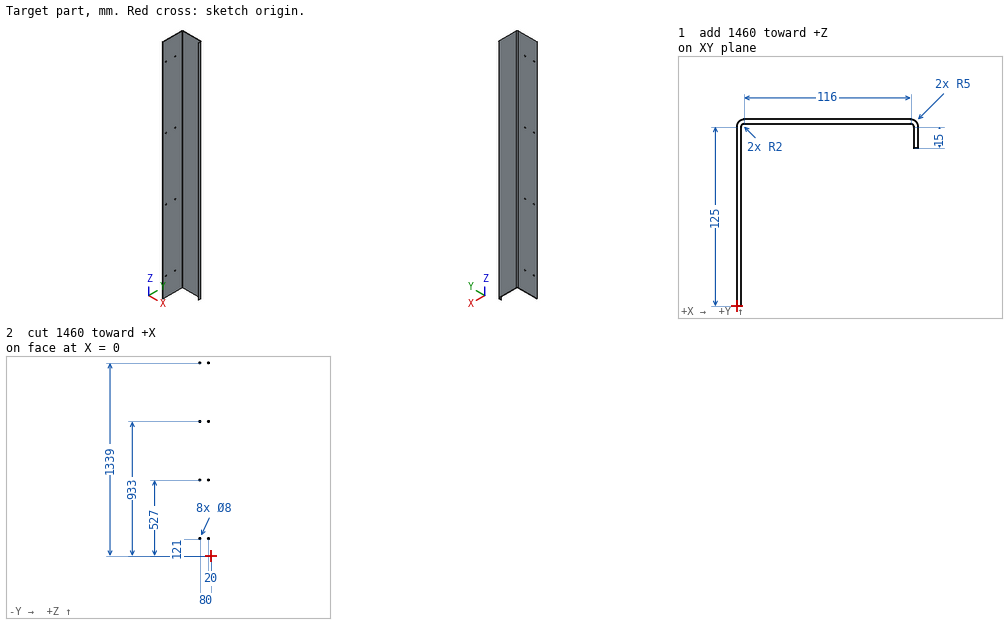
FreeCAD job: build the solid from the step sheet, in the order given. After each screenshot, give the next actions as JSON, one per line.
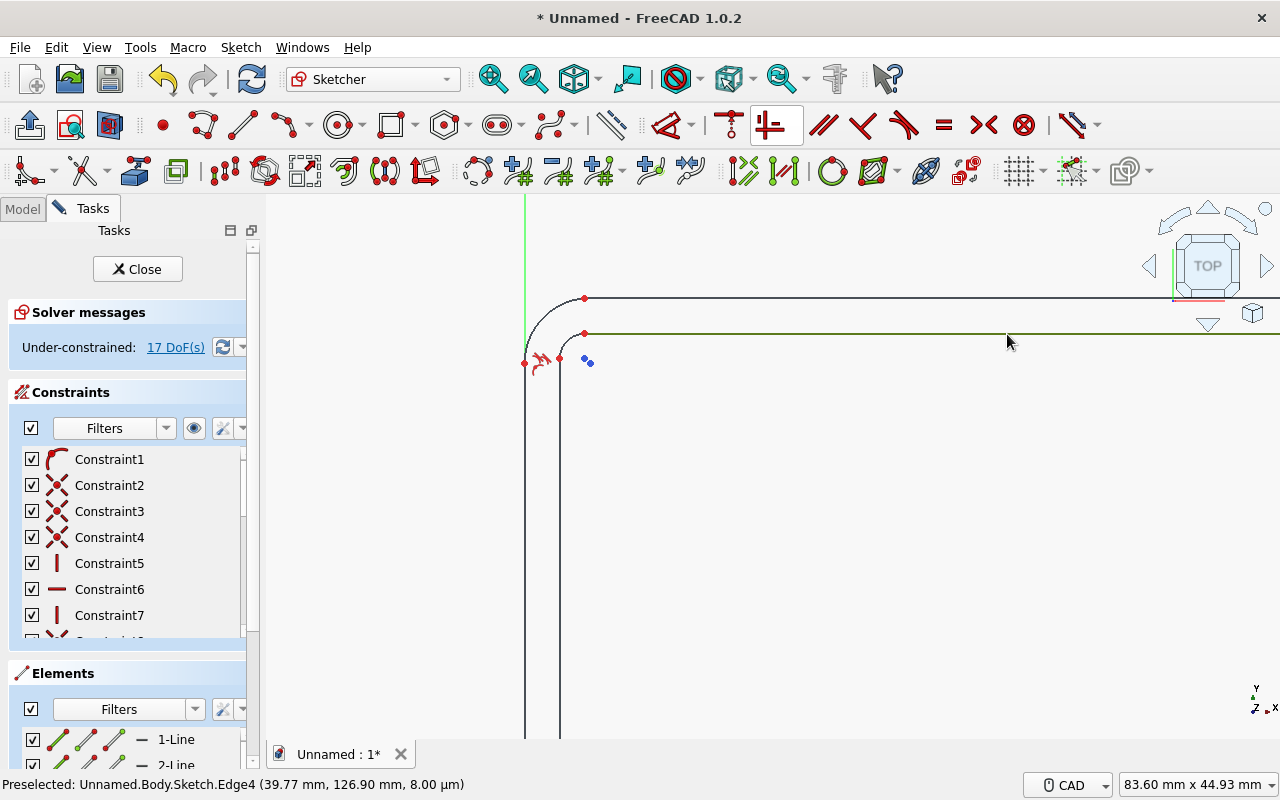
{"action": "left_click", "coordinate": [573, 337]}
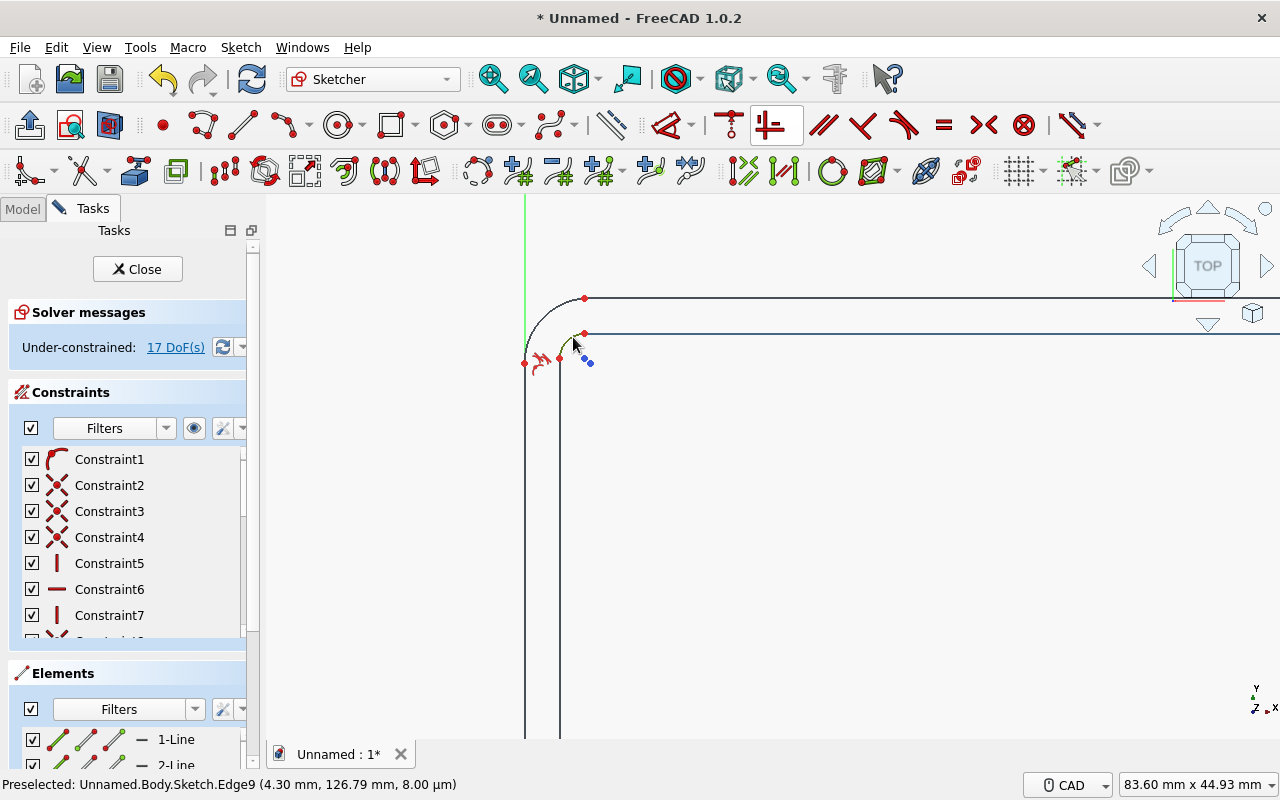
{"action": "left_click", "coordinate": [904, 126]}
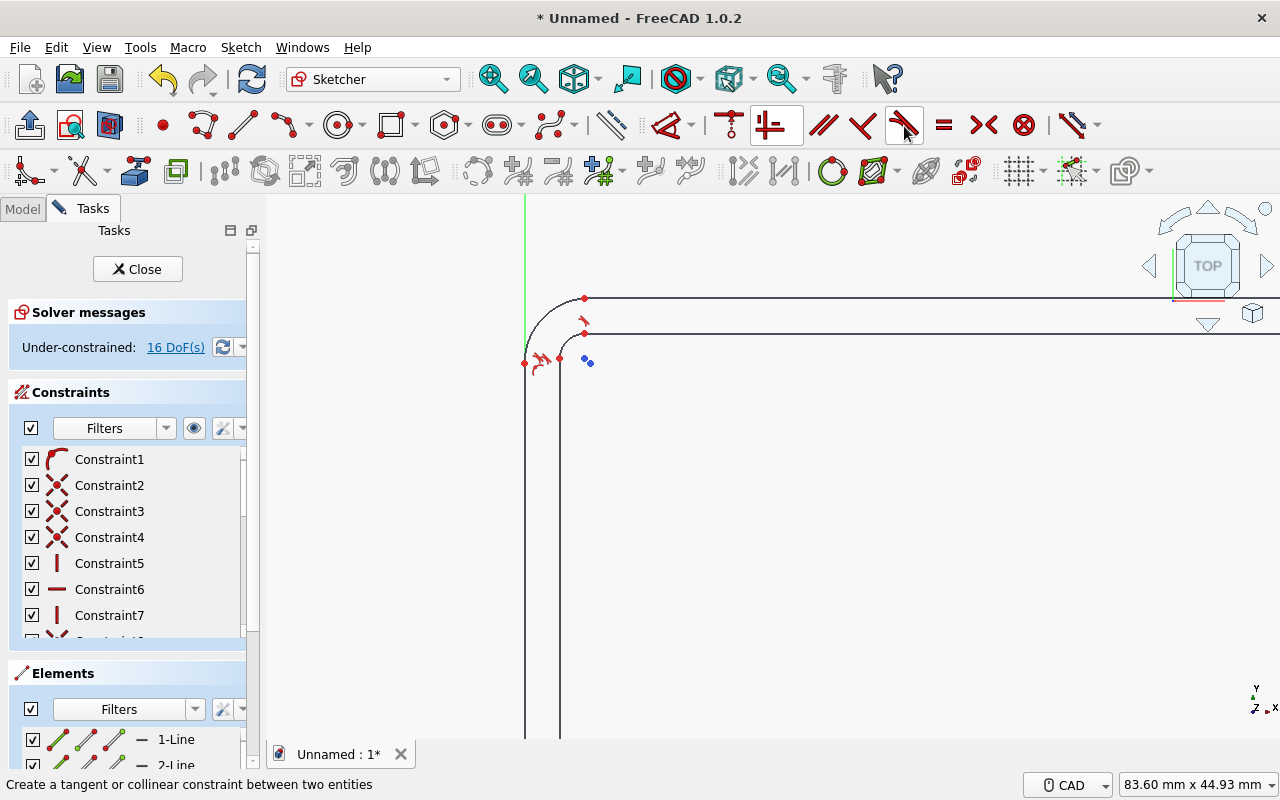
{"action": "left_click", "coordinate": [1007, 334]}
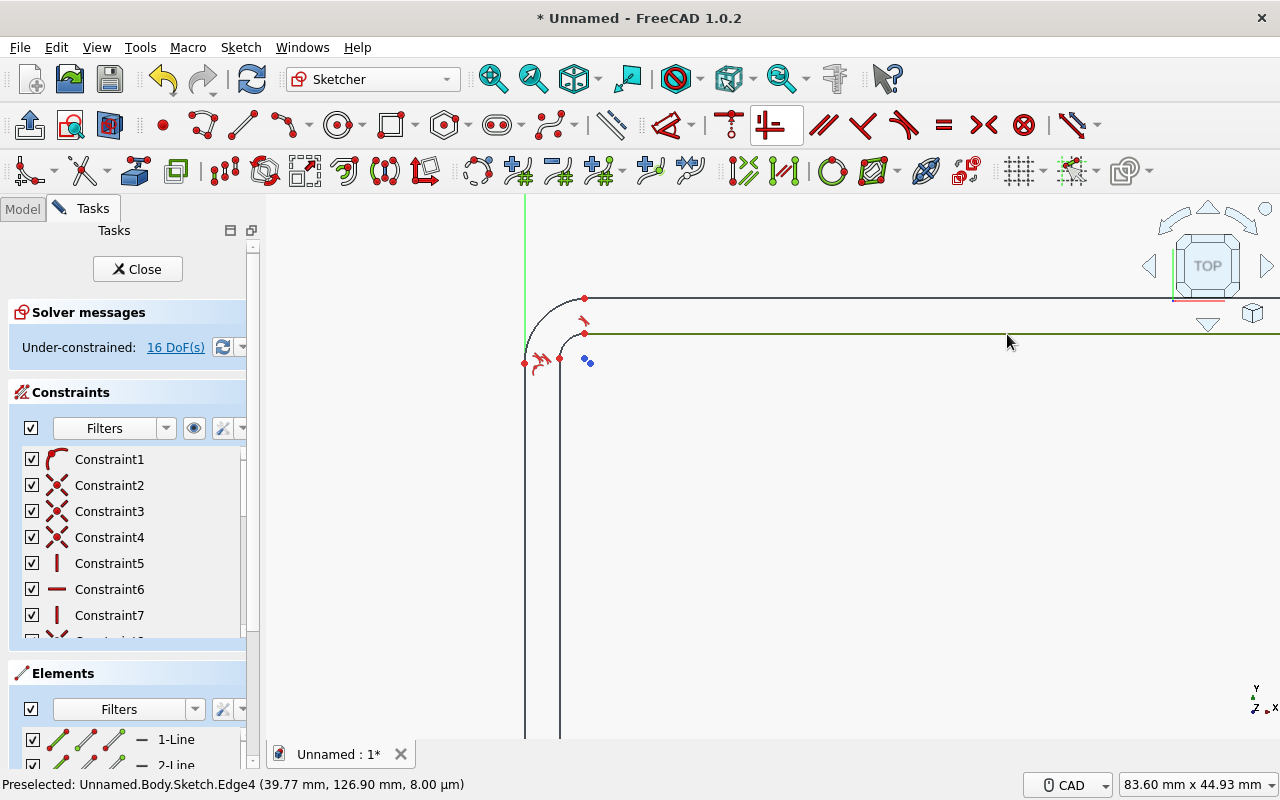
{"action": "scroll", "coordinate": [557, 310], "scroll_direction": "down", "scroll_amount": 8}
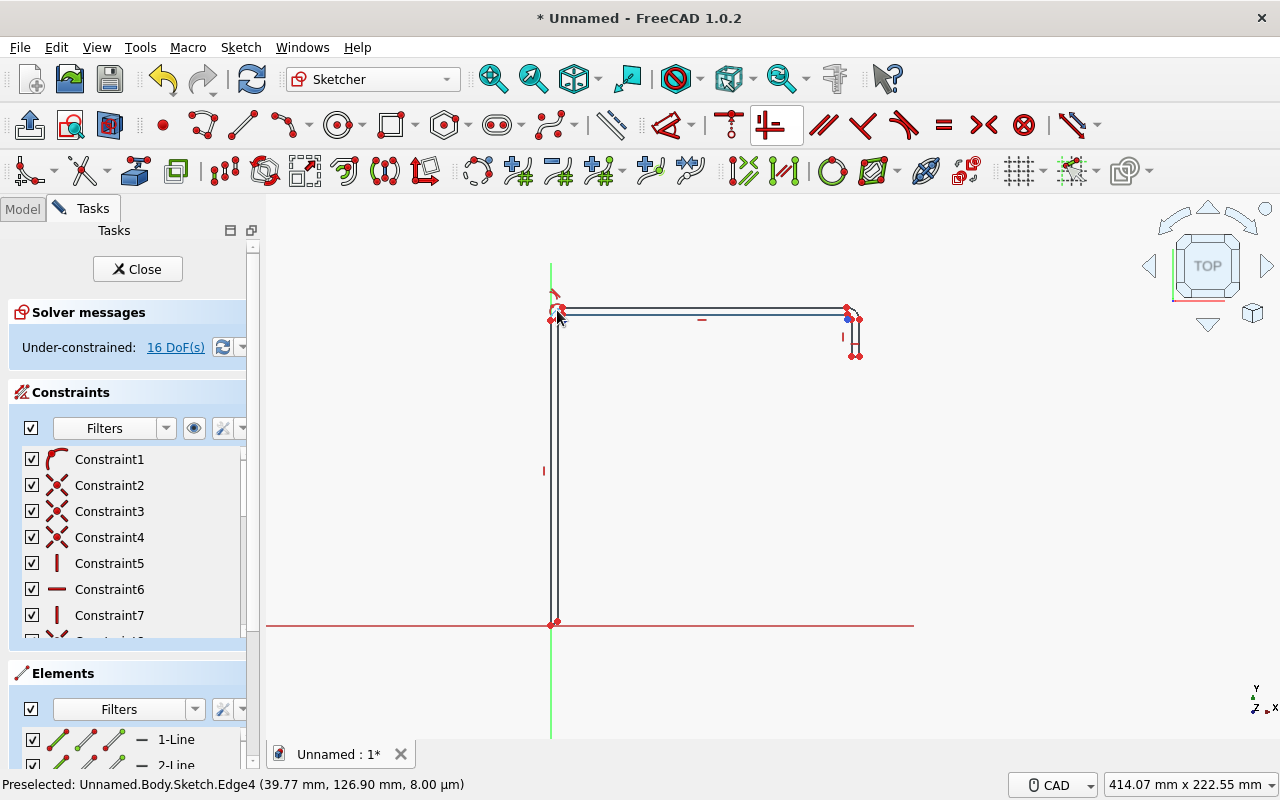
{"action": "scroll", "coordinate": [851, 318], "scroll_direction": "up", "scroll_amount": 9}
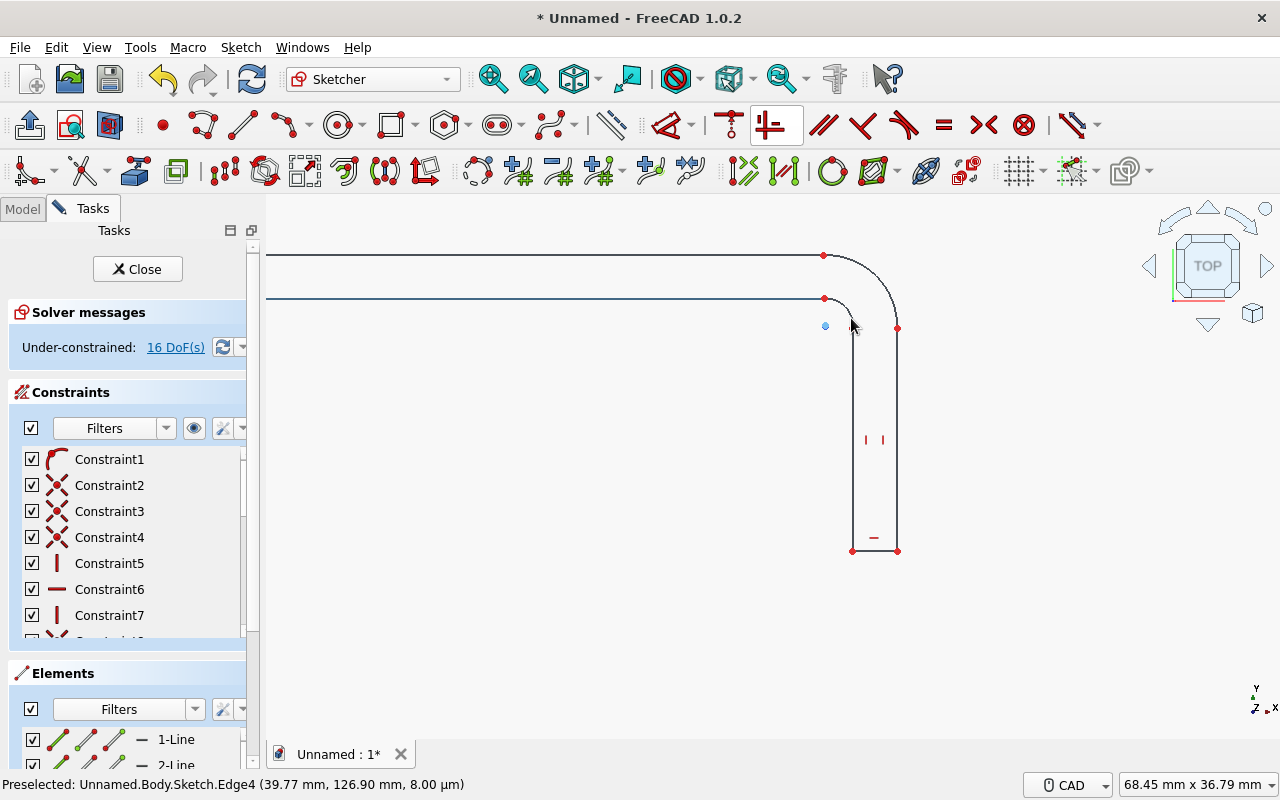
{"action": "left_click", "coordinate": [851, 315]}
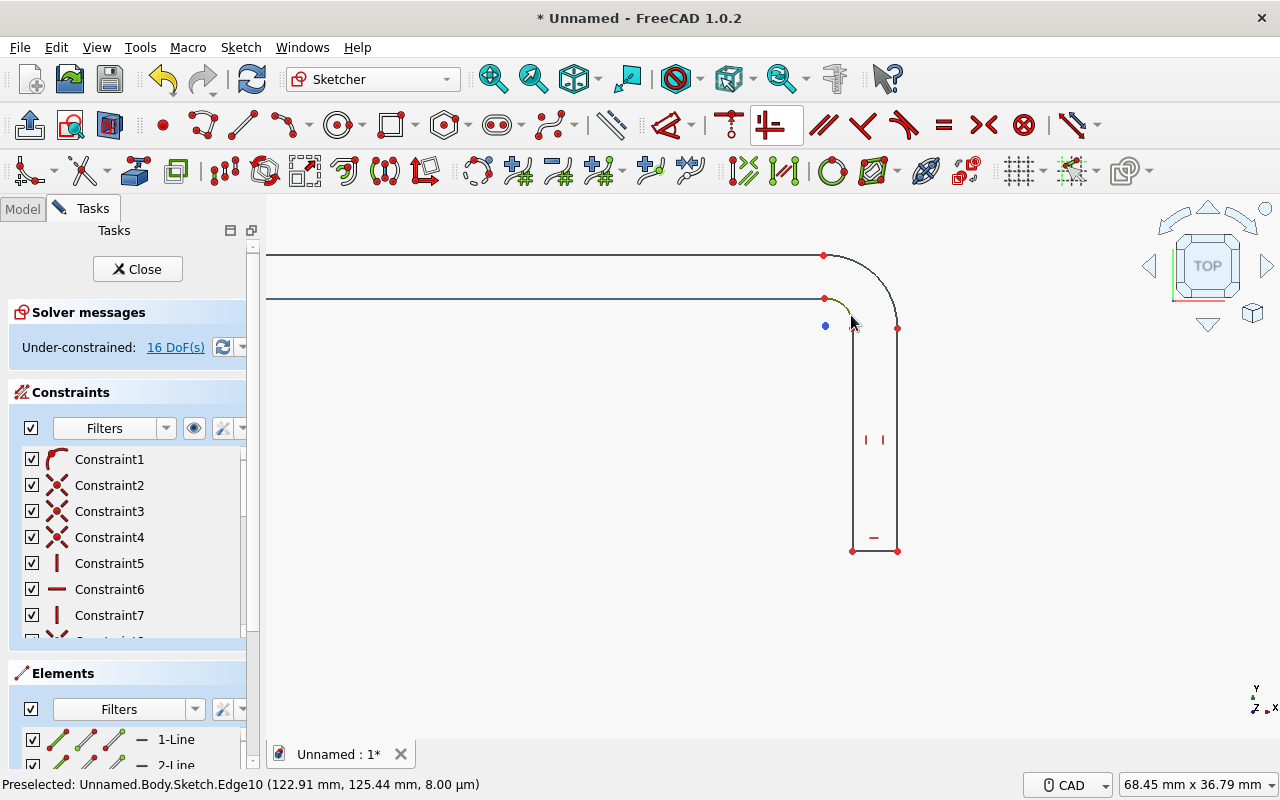
{"action": "left_click", "coordinate": [904, 126]}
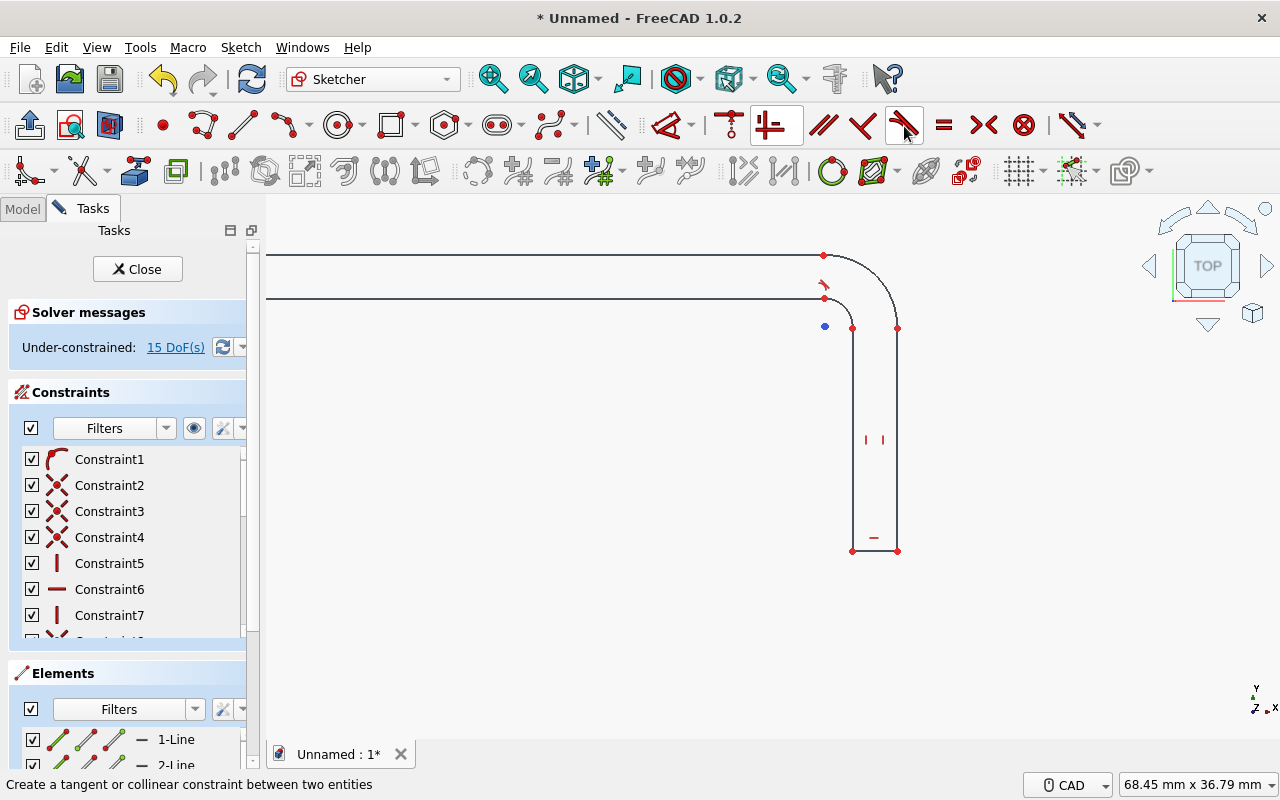
{"action": "scroll", "coordinate": [851, 318], "scroll_direction": "down", "scroll_amount": 9}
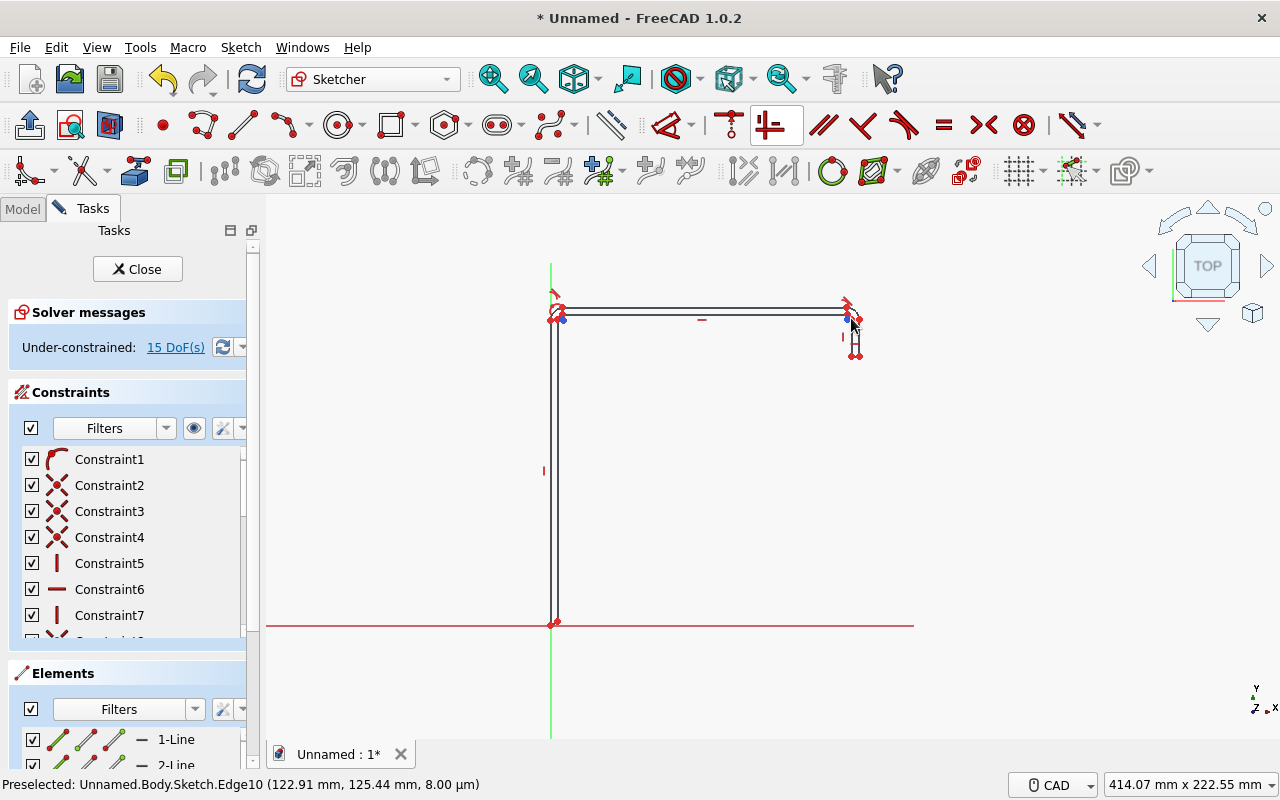
{"action": "scroll", "coordinate": [852, 331], "scroll_direction": "up", "scroll_amount": 4}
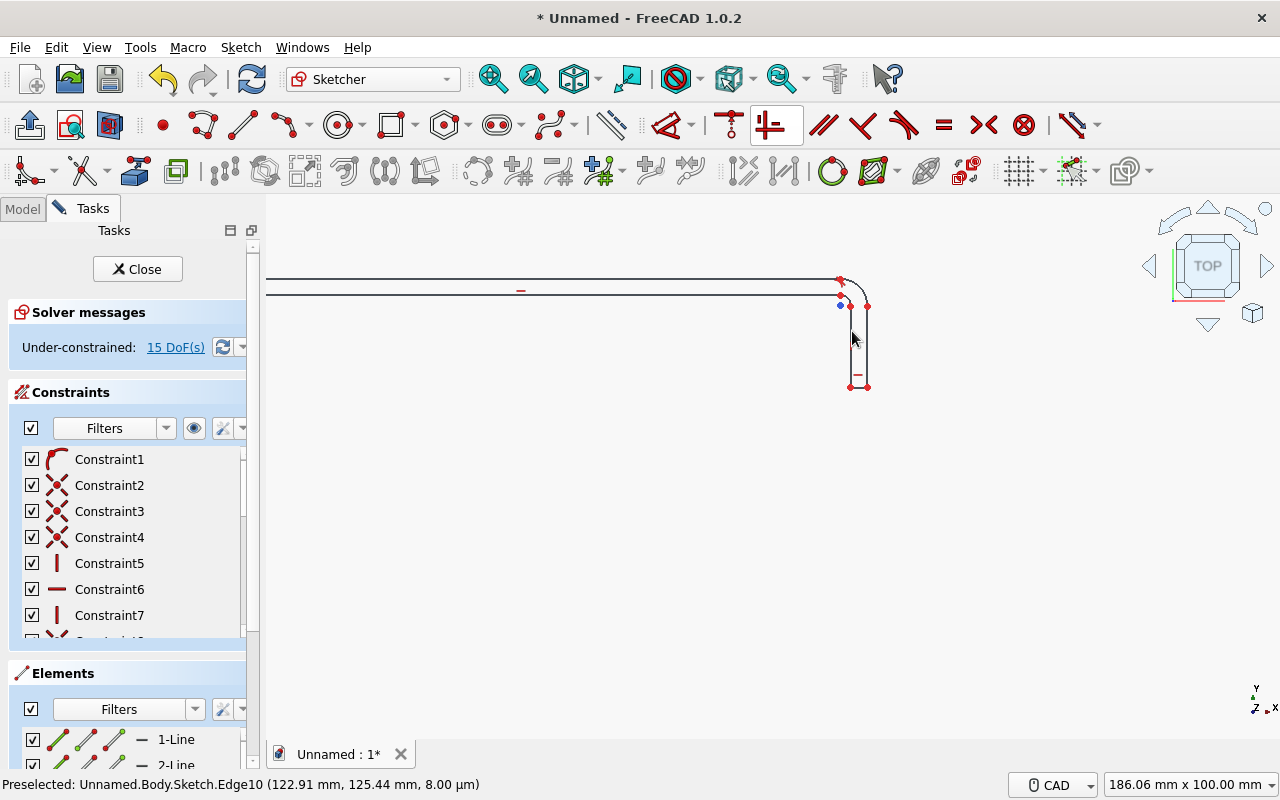
{"action": "left_click", "coordinate": [851, 331]}